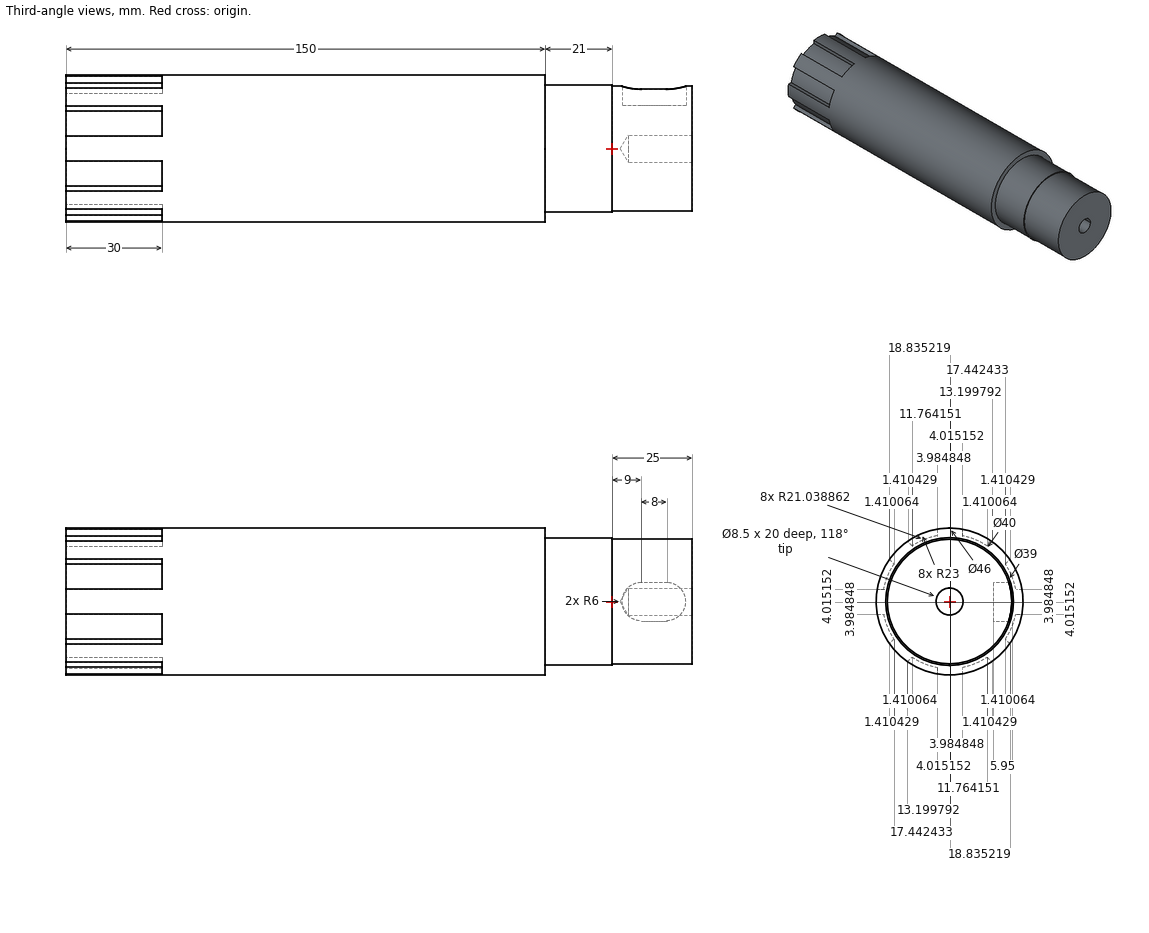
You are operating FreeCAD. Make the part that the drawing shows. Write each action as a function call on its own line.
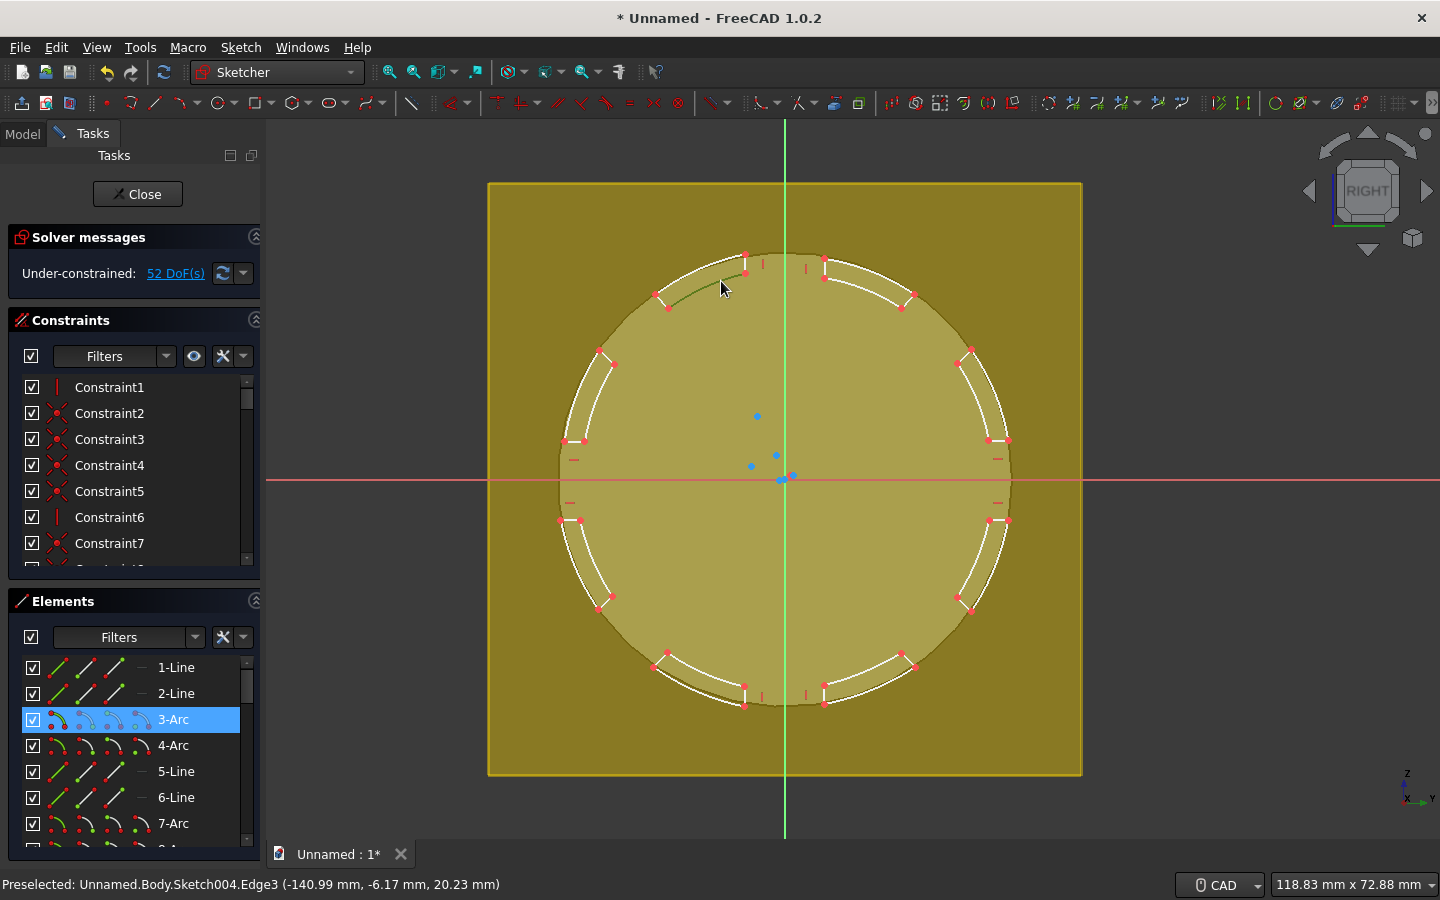
click(1002, 412)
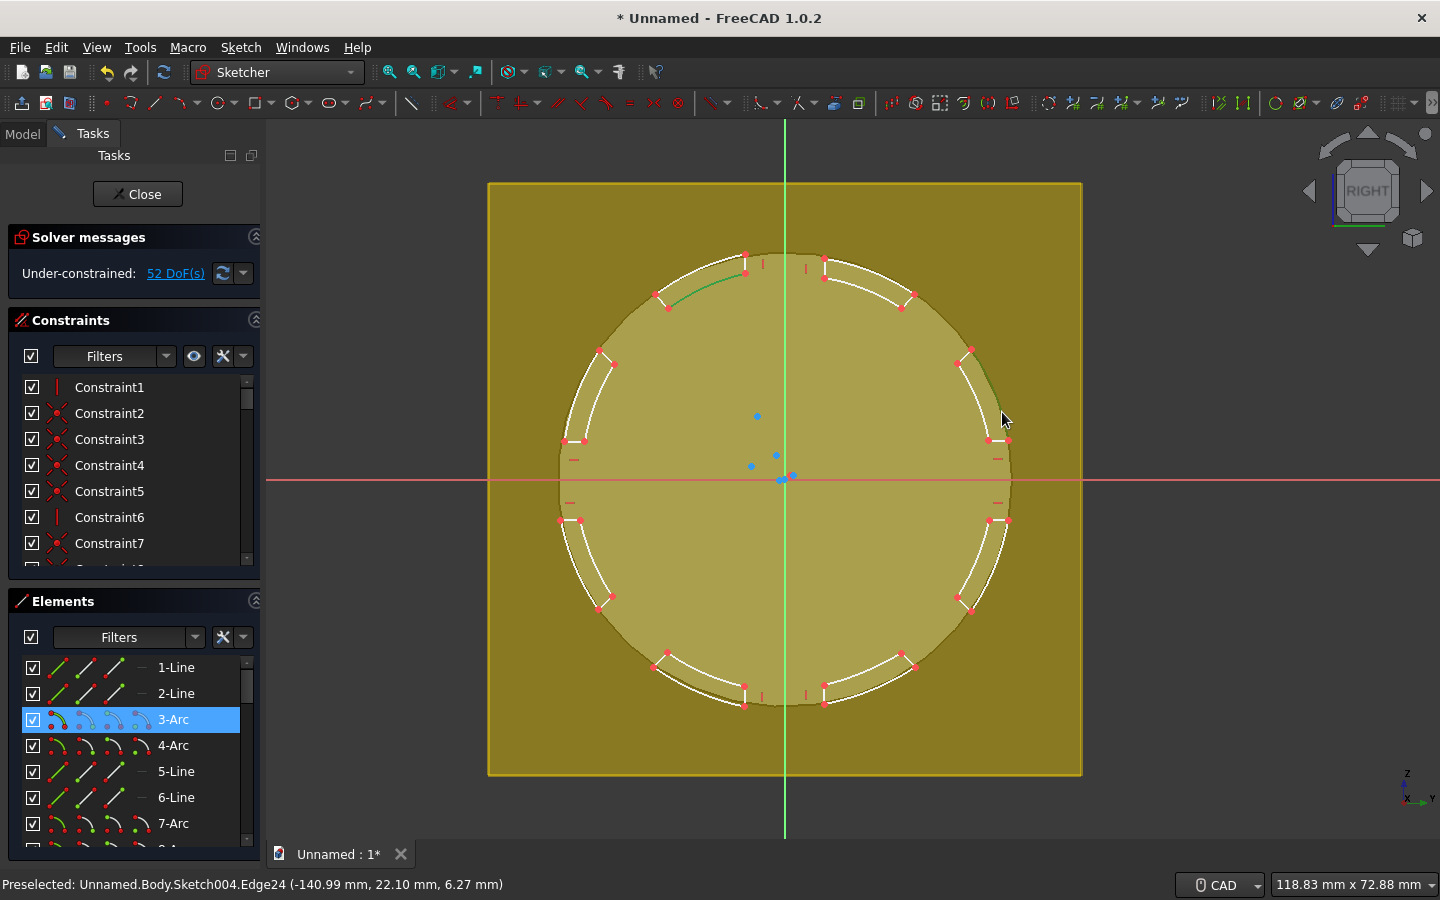
click(498, 104)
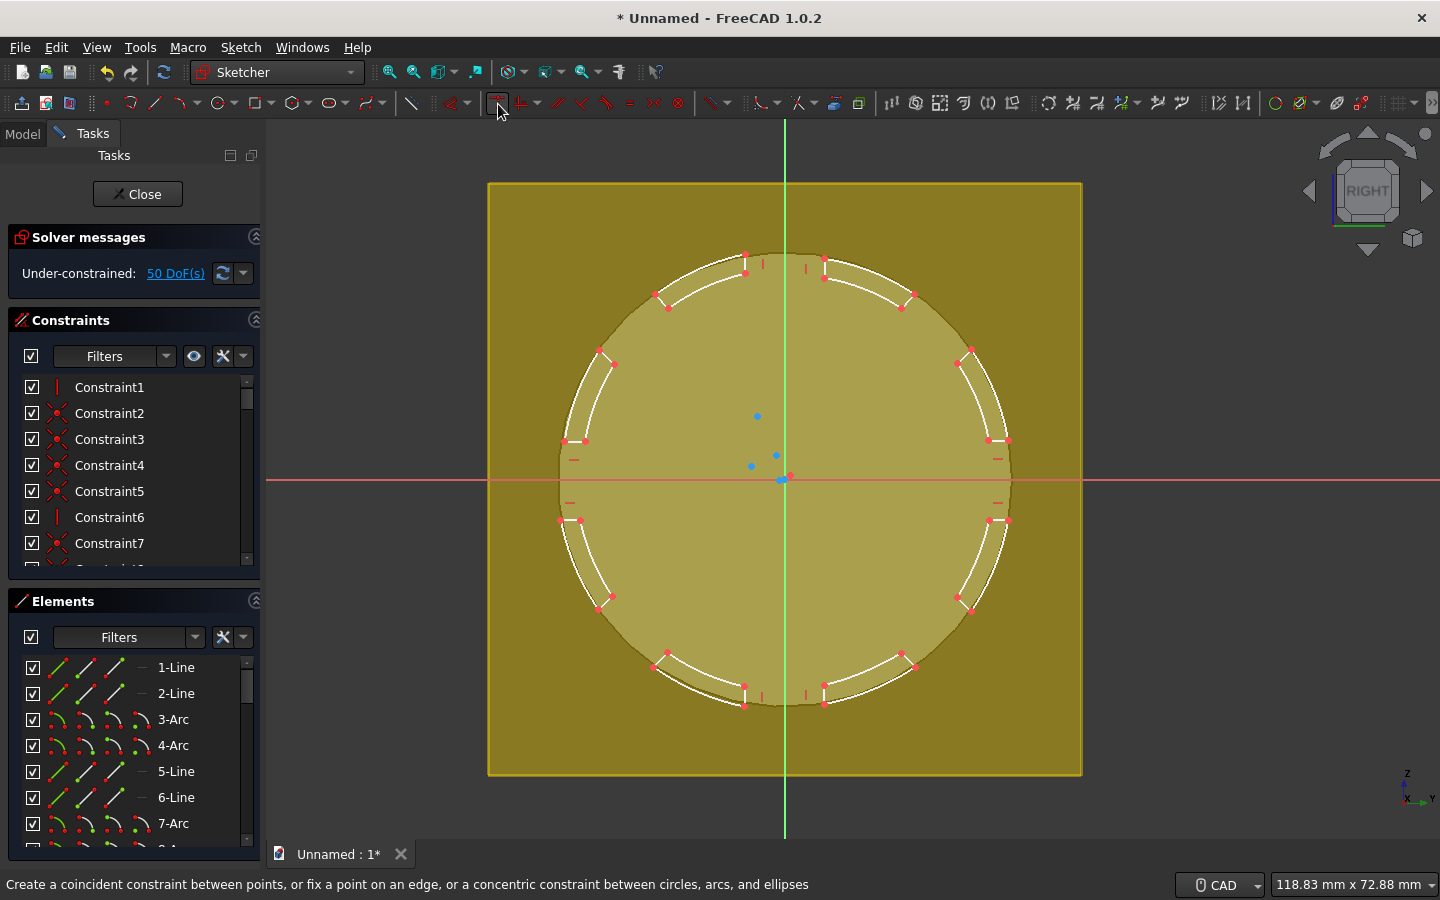
click(721, 281)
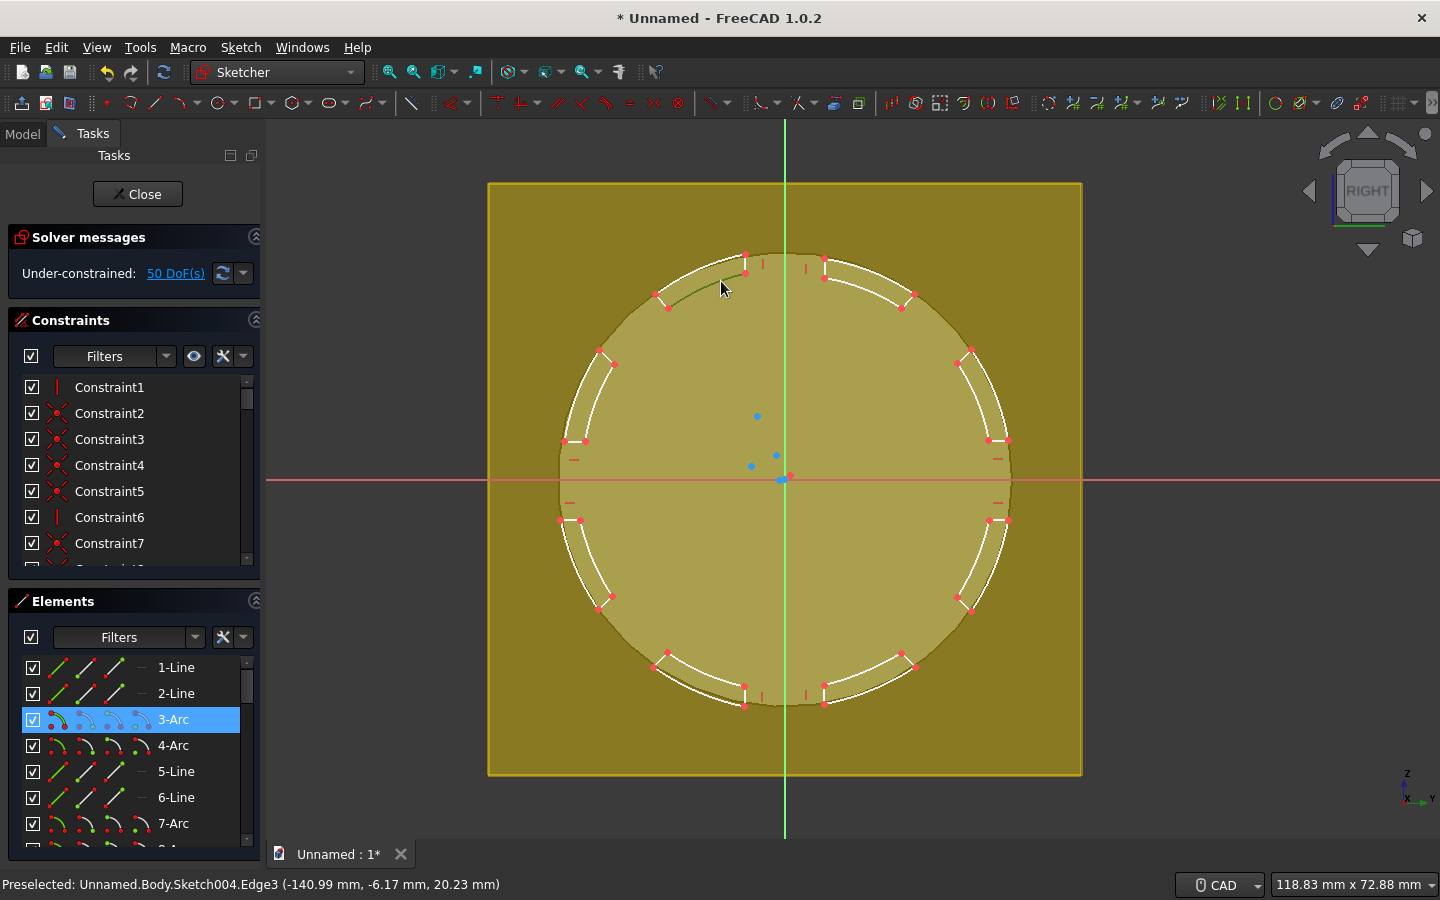
click(986, 586)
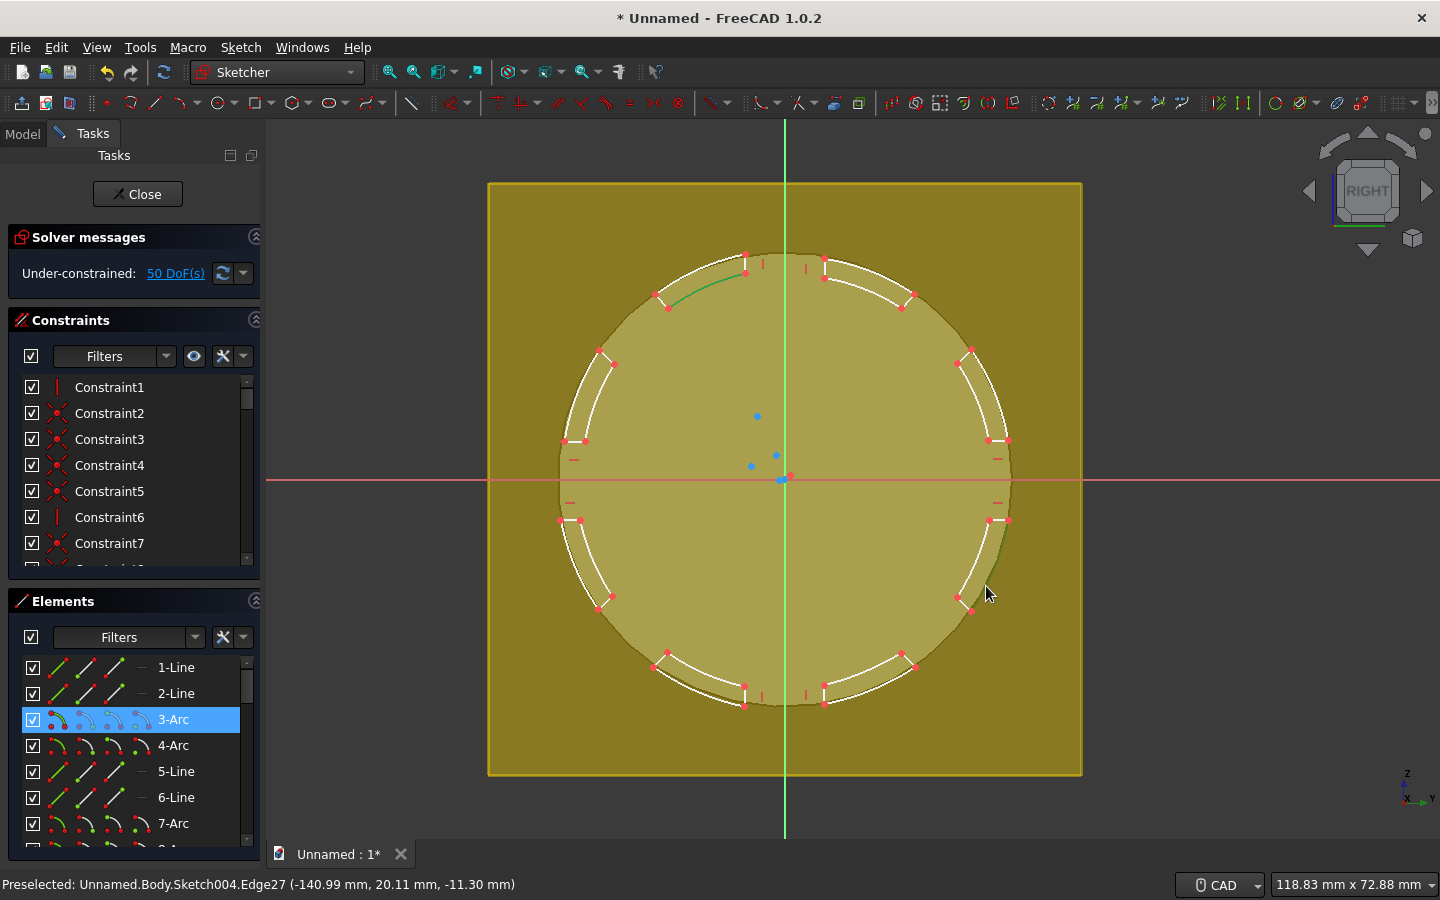
click(498, 104)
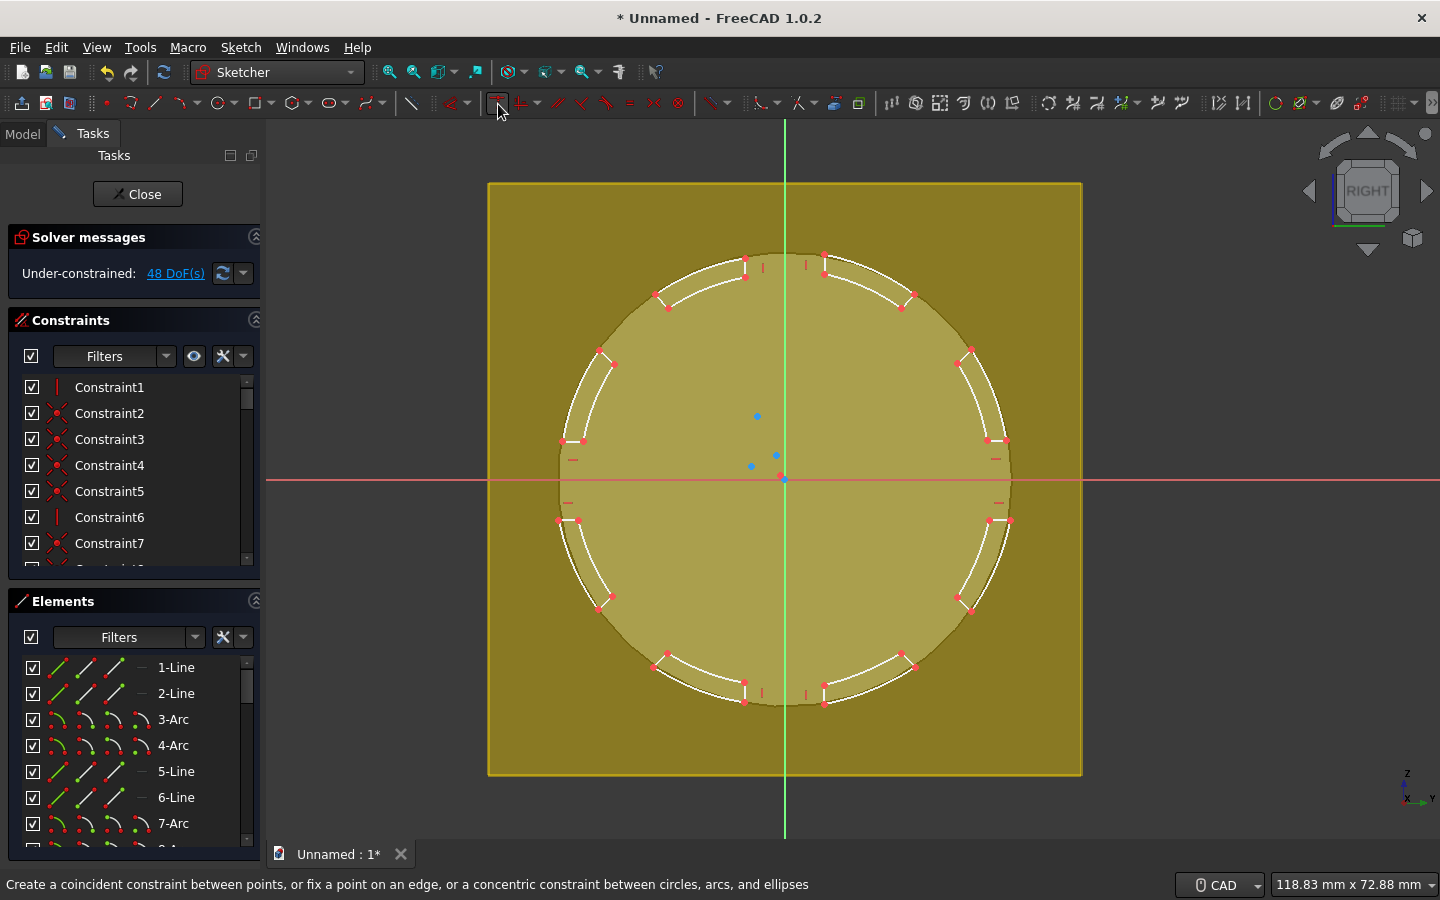
click(721, 283)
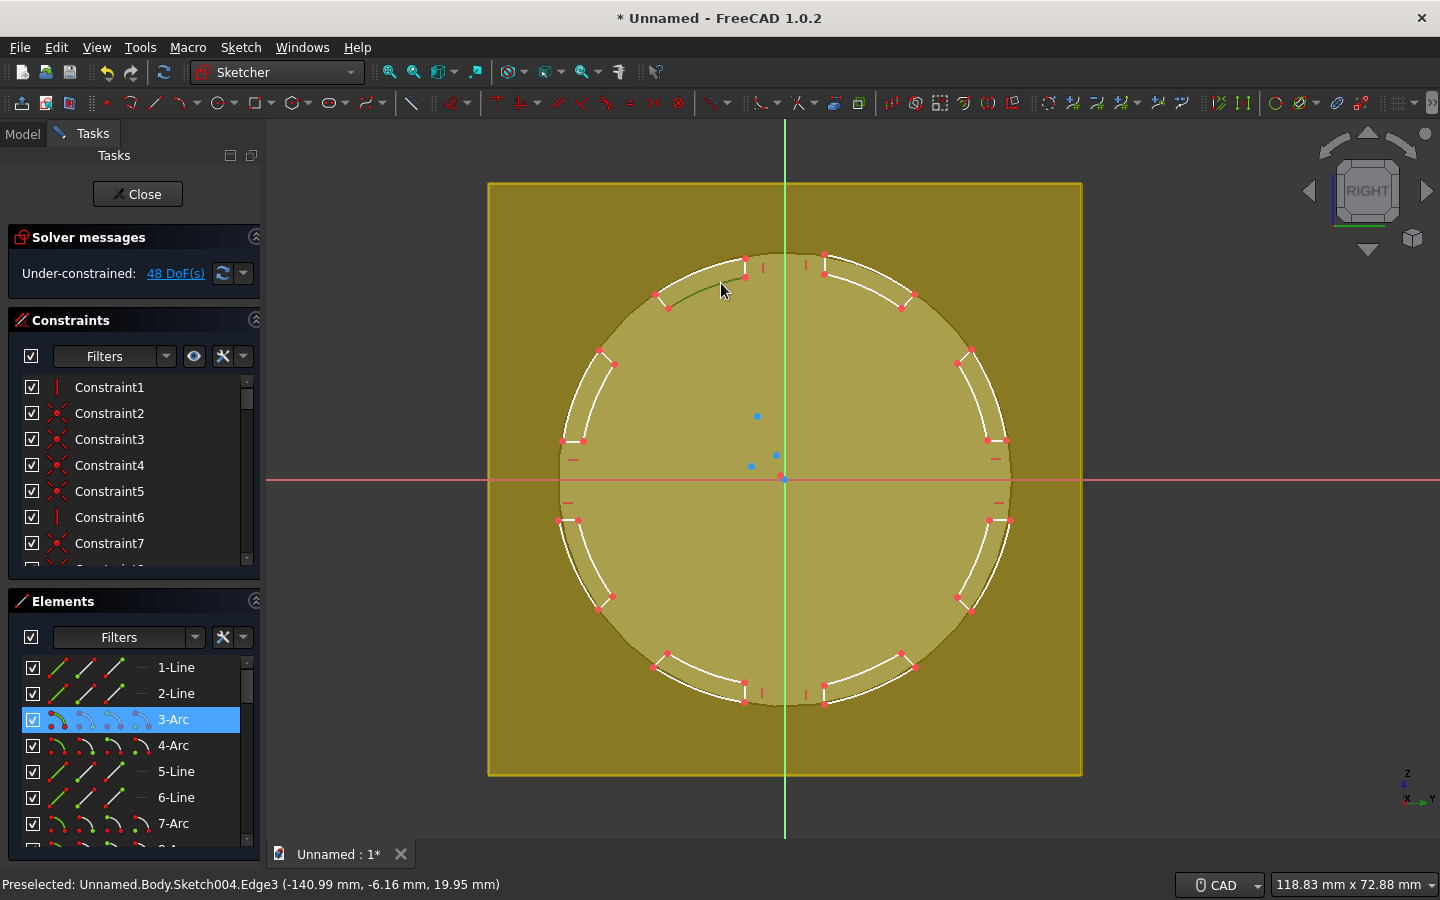
click(970, 576)